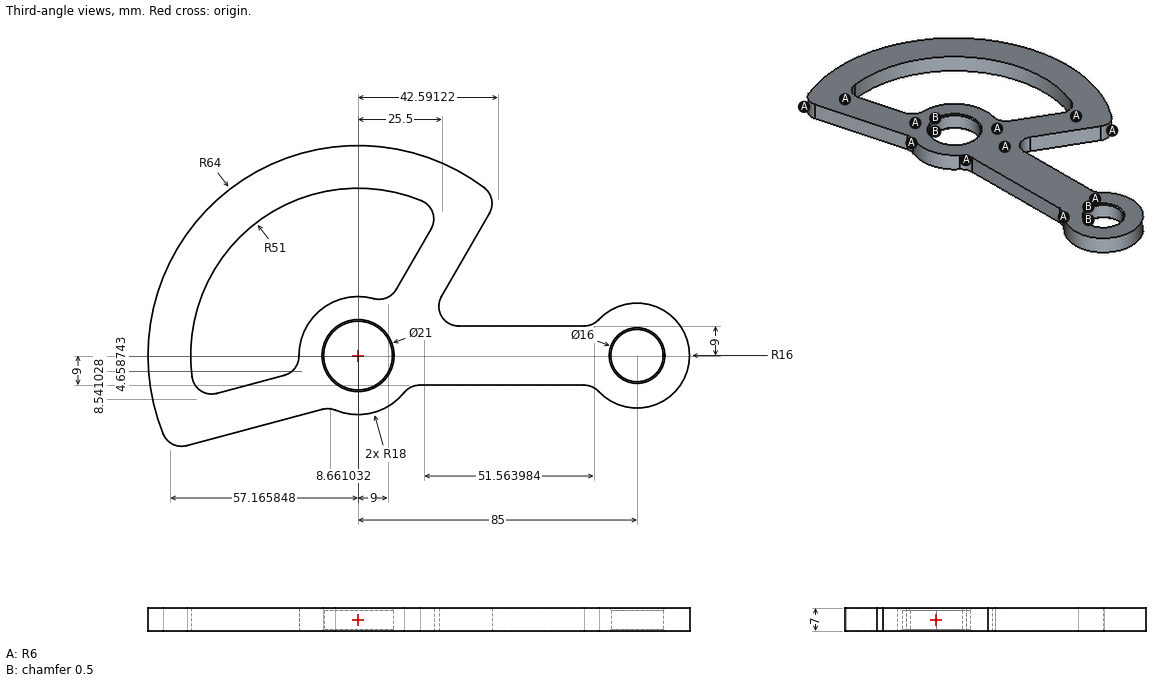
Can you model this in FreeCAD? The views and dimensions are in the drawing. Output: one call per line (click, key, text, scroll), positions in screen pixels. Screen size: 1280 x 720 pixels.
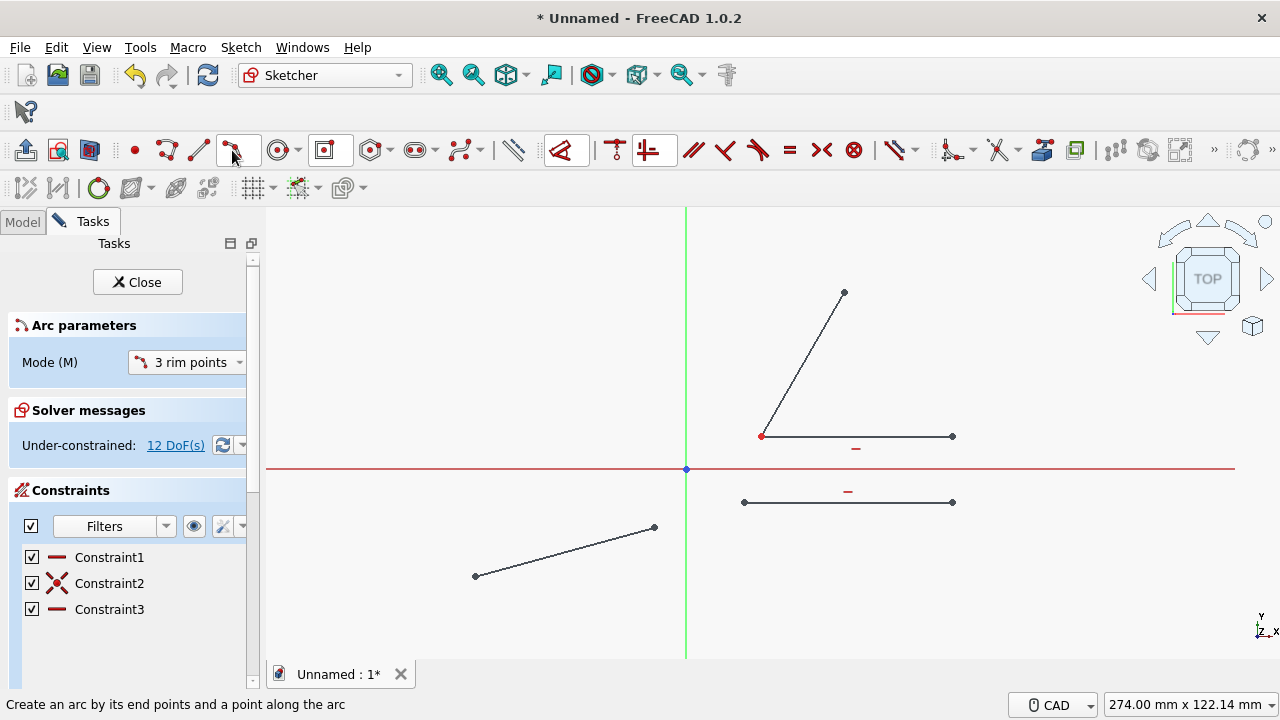
click(844, 293)
click(475, 577)
click(542, 281)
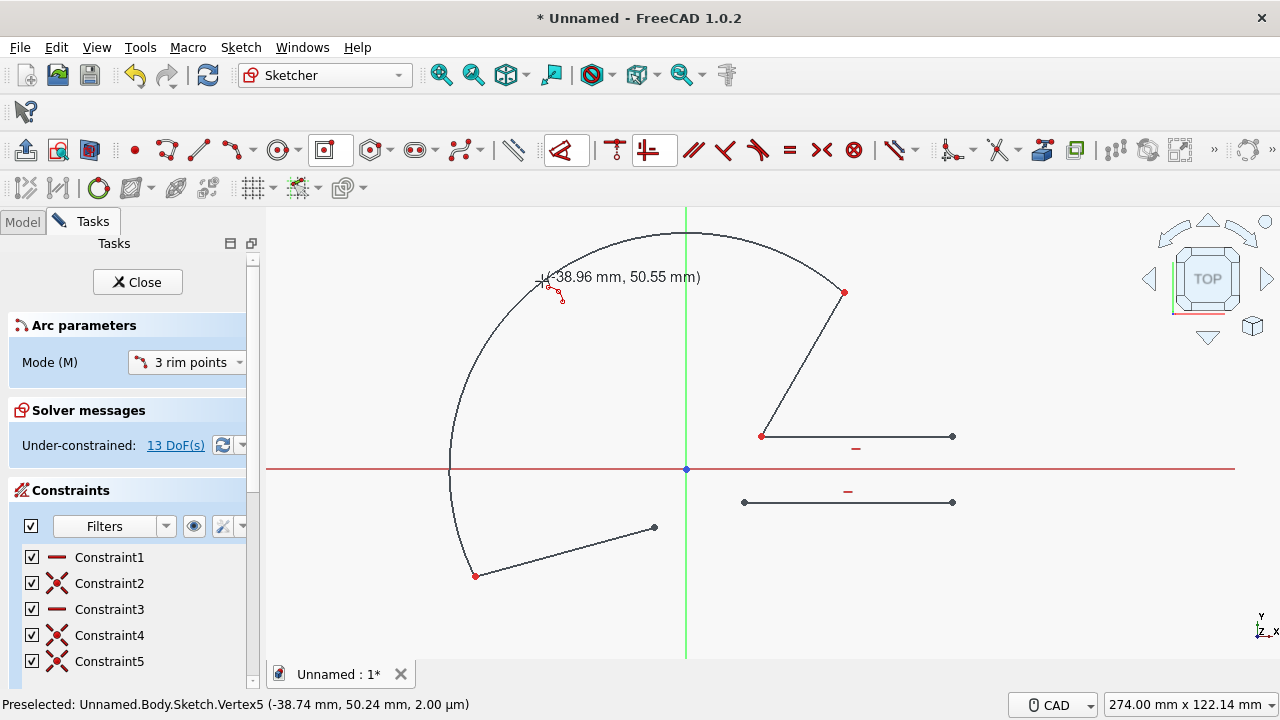
click(654, 528)
click(744, 503)
click(704, 533)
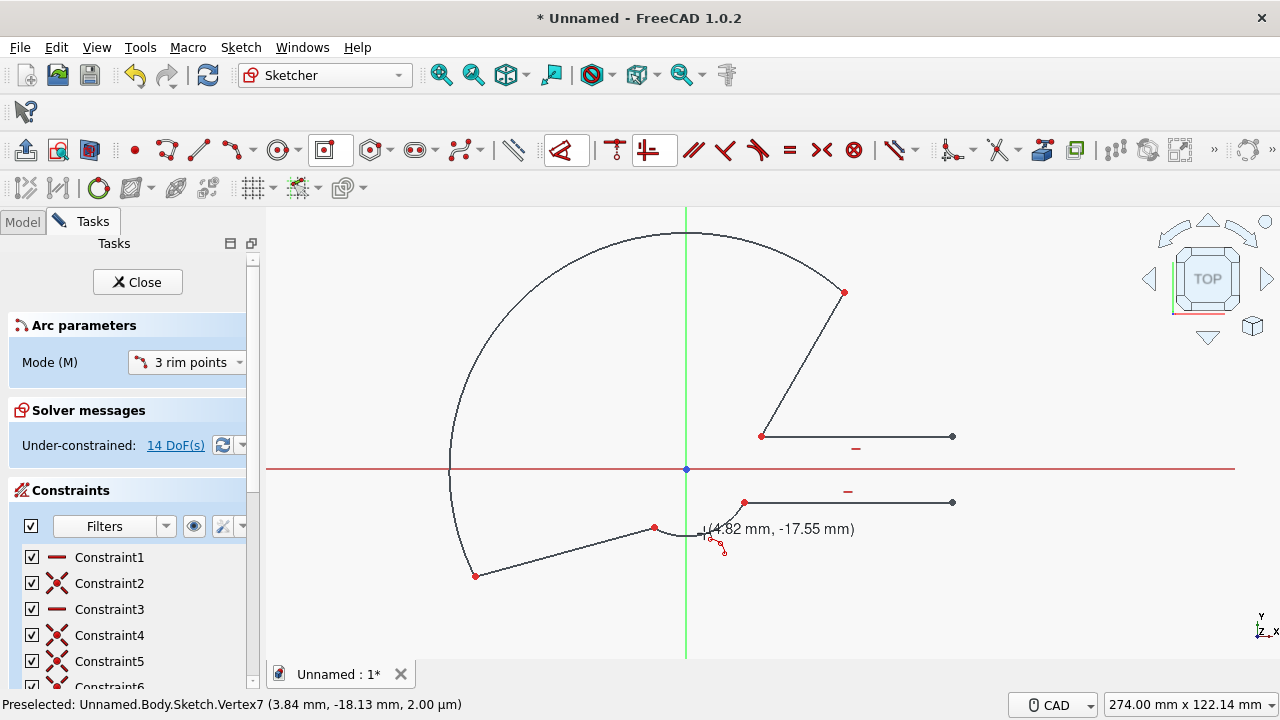
click(952, 503)
click(952, 437)
click(1052, 498)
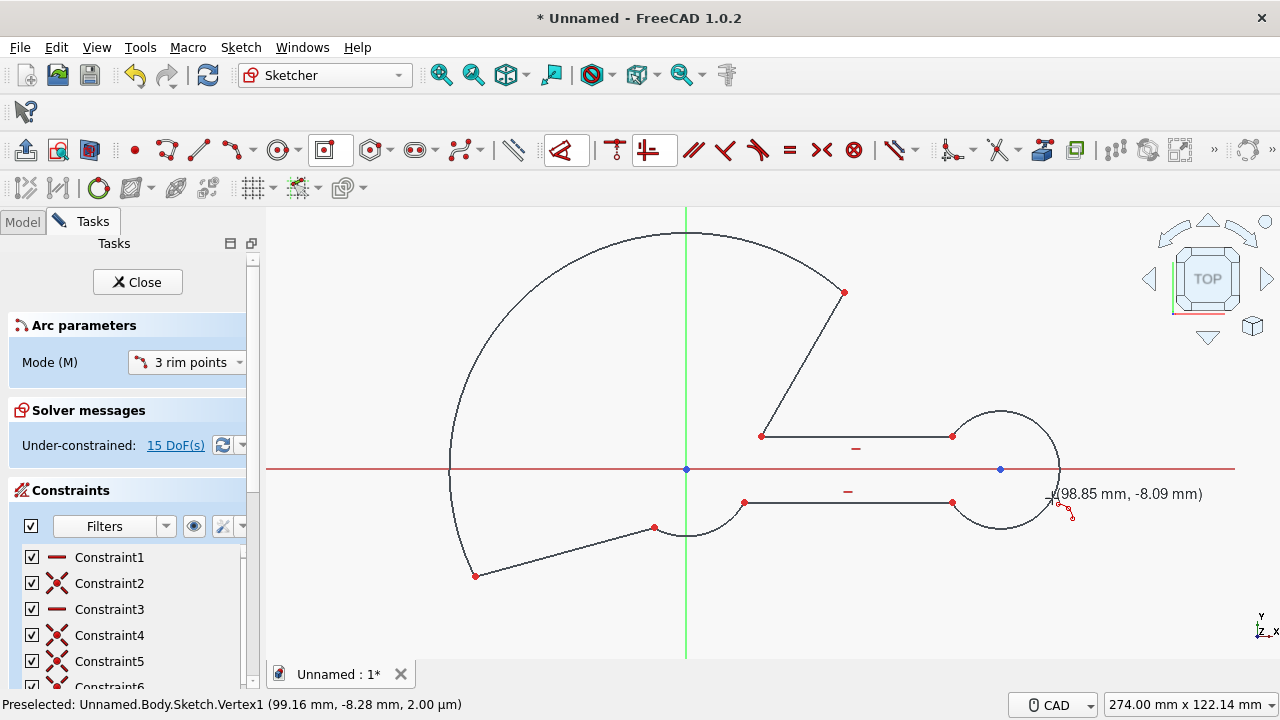
click(200, 150)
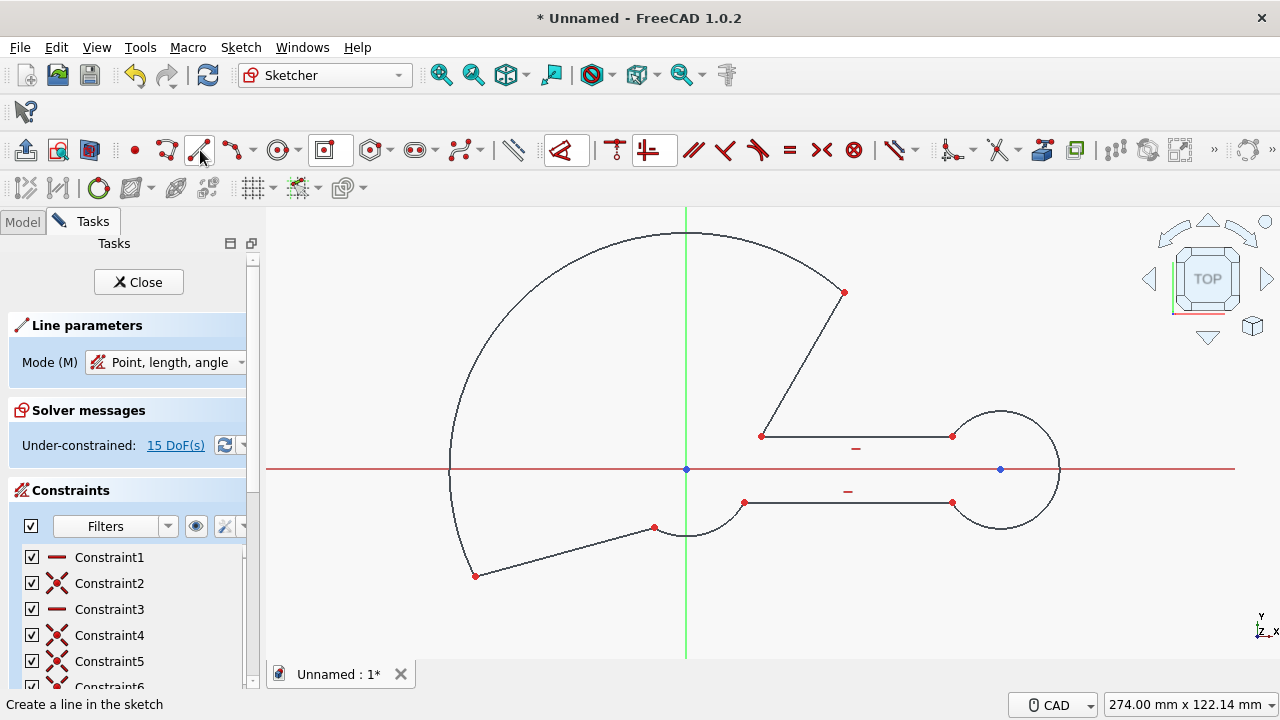
click(622, 486)
click(504, 518)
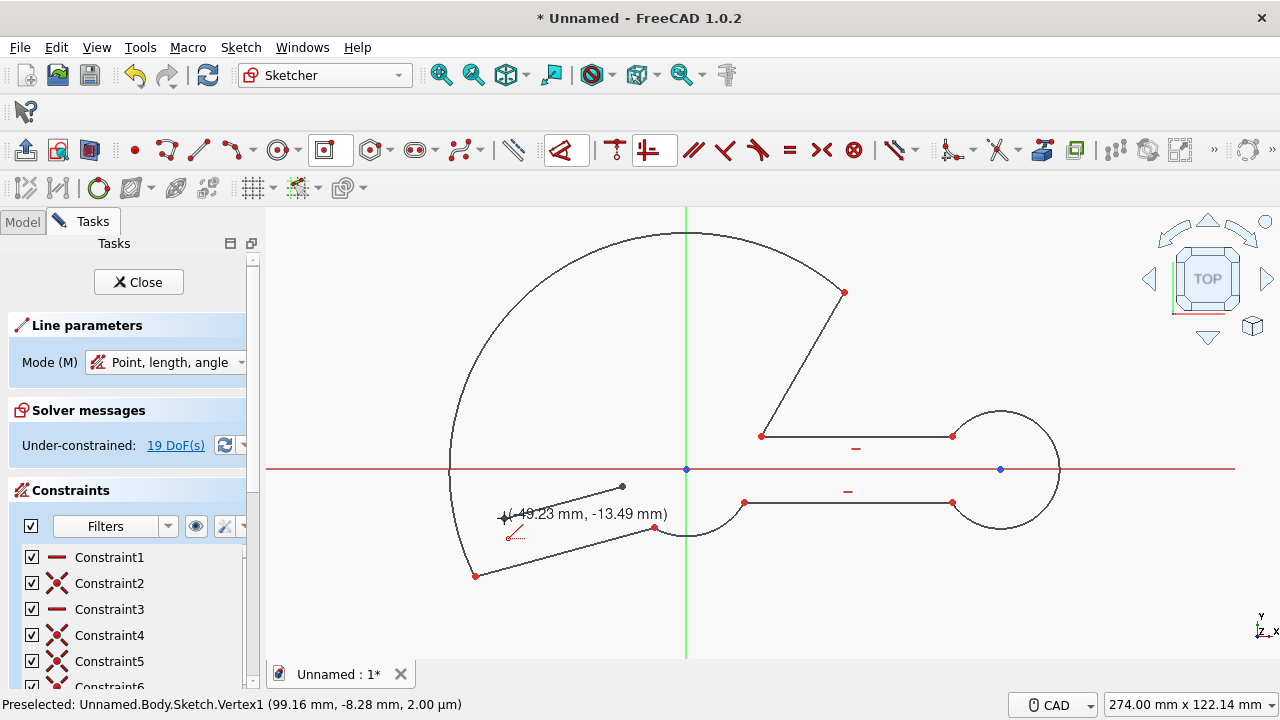
click(781, 306)
click(719, 411)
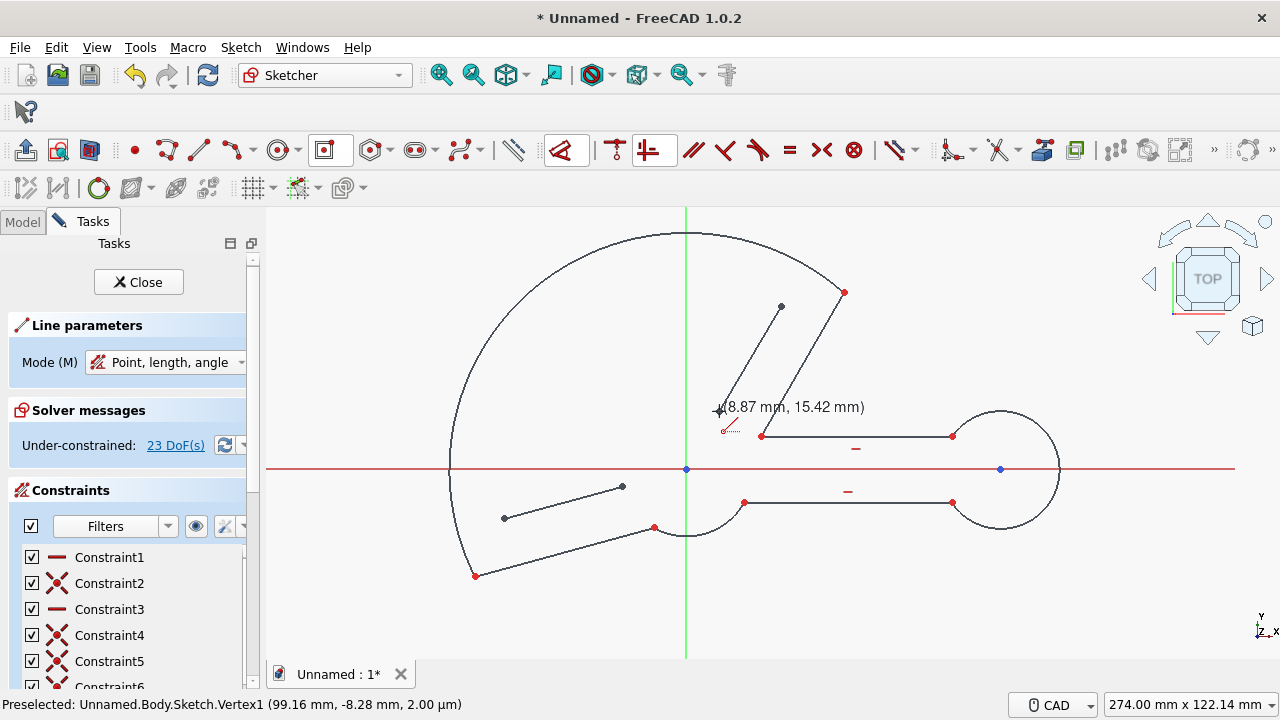
click(232, 150)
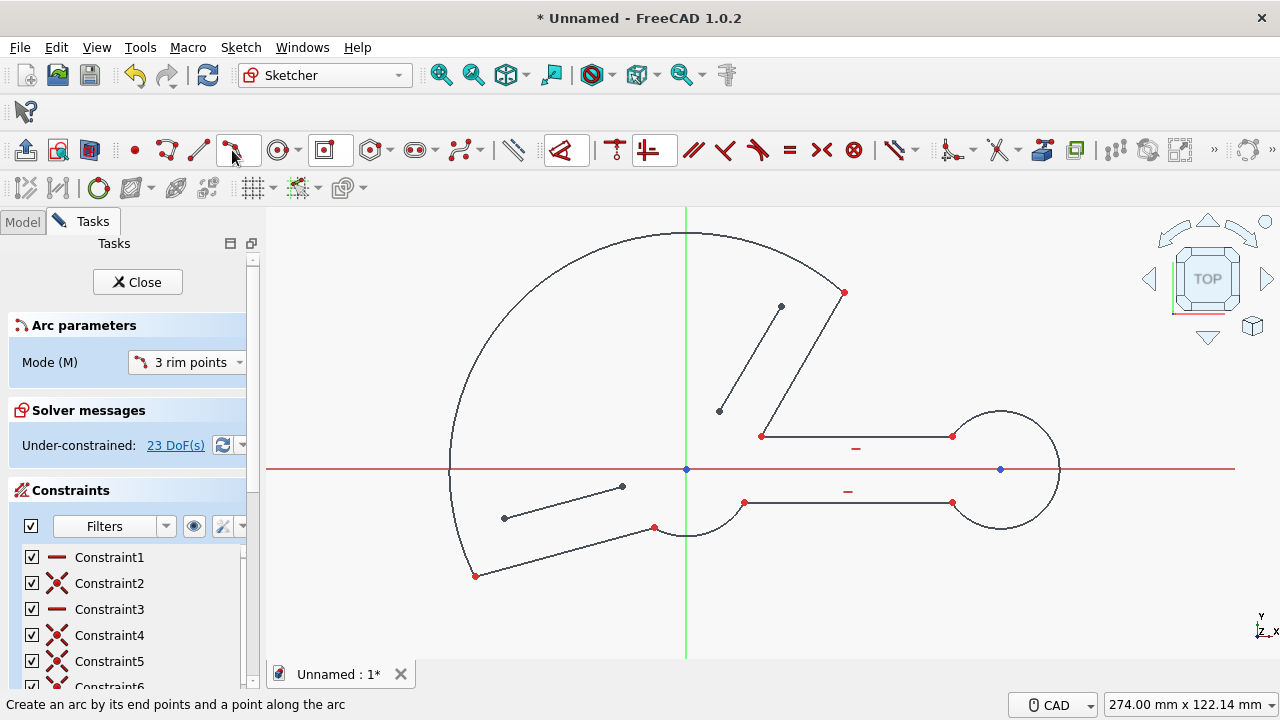
click(504, 519)
click(781, 307)
click(571, 319)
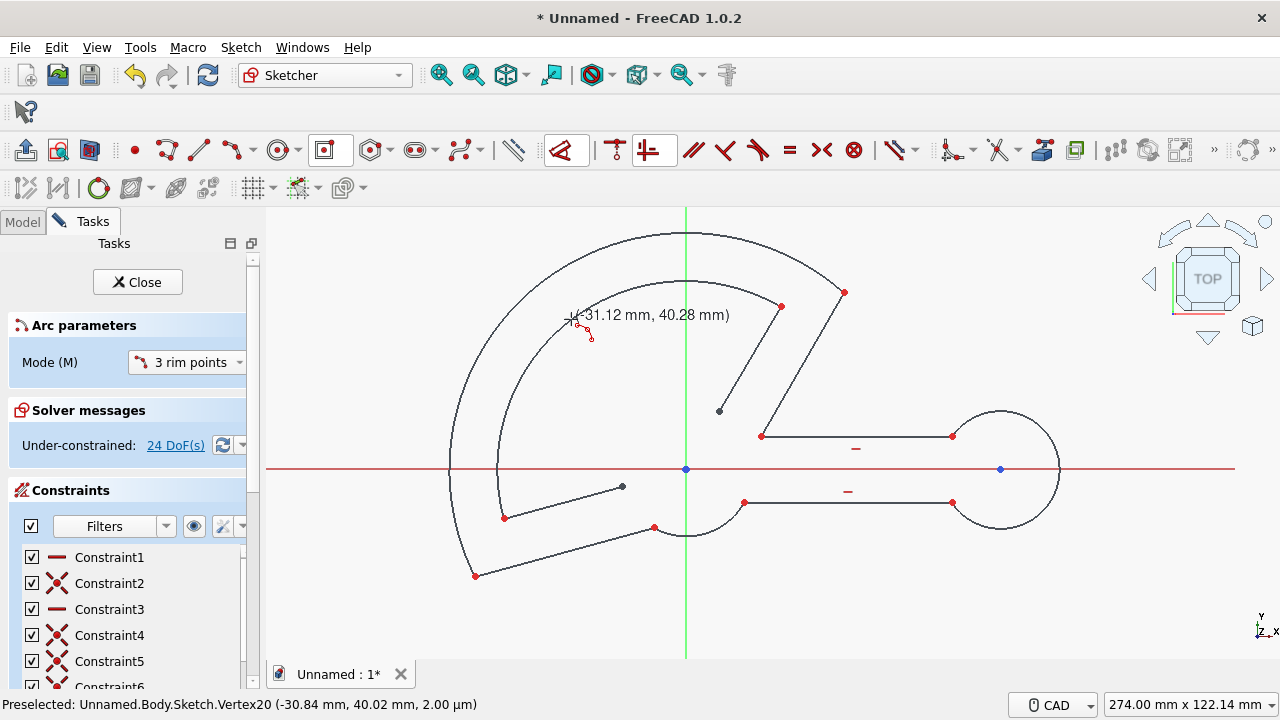
click(719, 412)
click(622, 487)
click(646, 416)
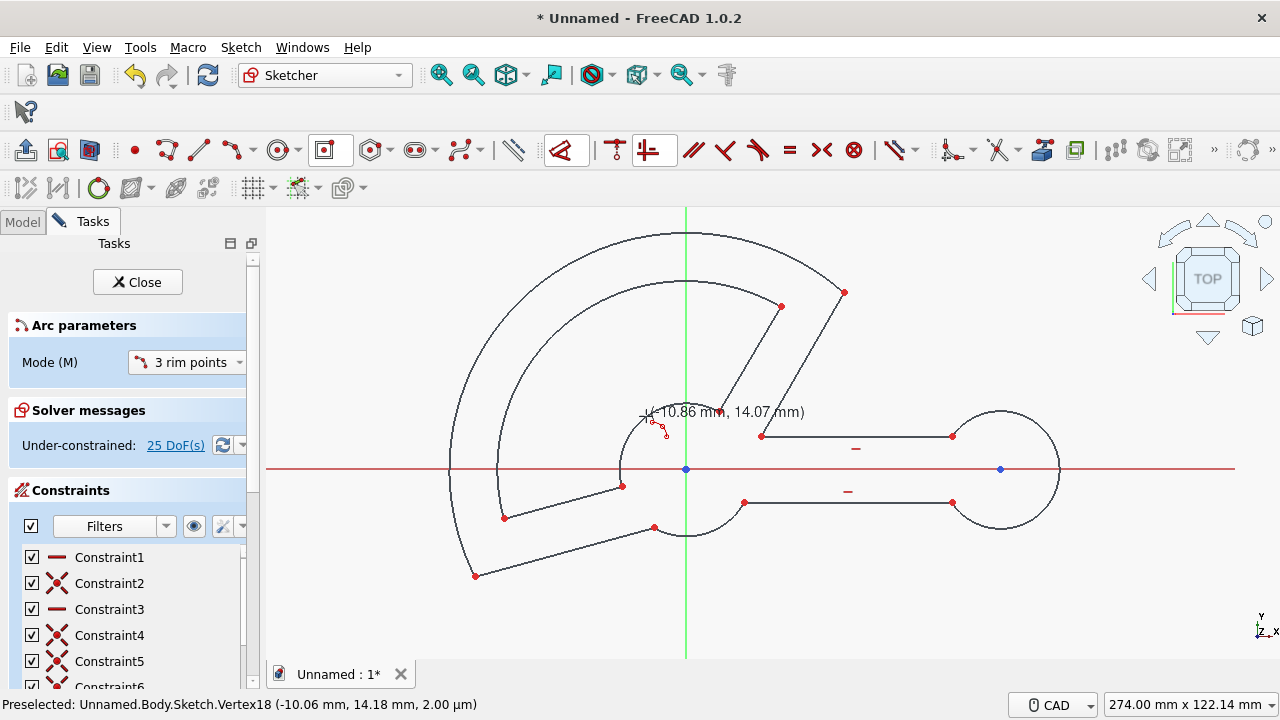
click(278, 150)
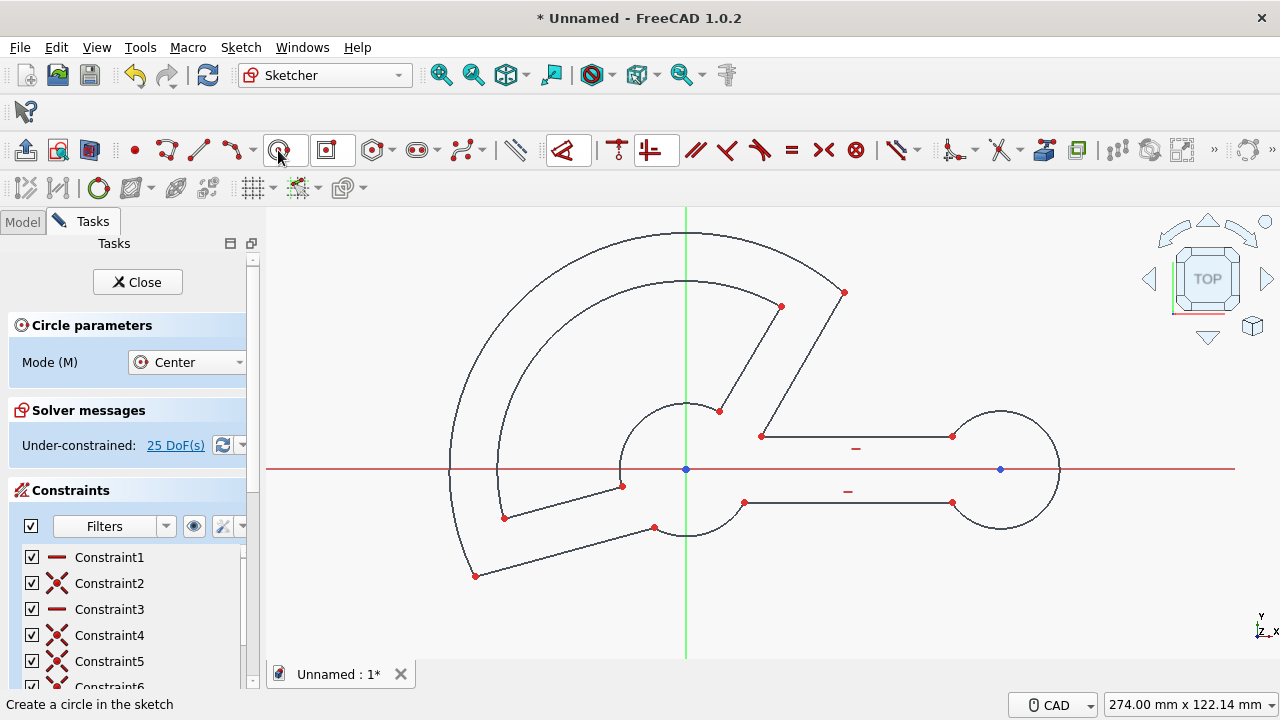
click(1001, 469)
move(1022, 448)